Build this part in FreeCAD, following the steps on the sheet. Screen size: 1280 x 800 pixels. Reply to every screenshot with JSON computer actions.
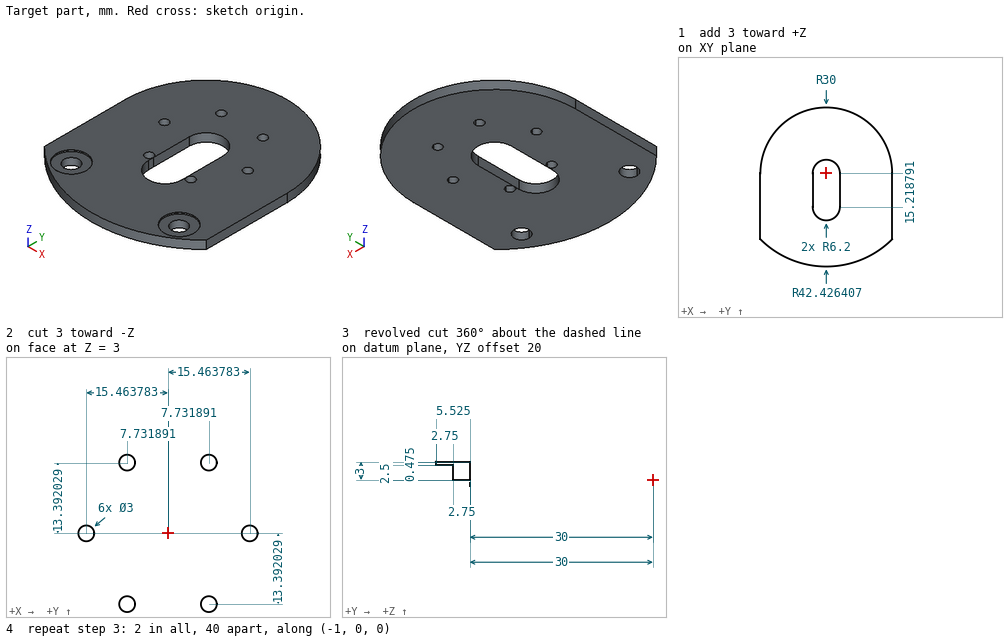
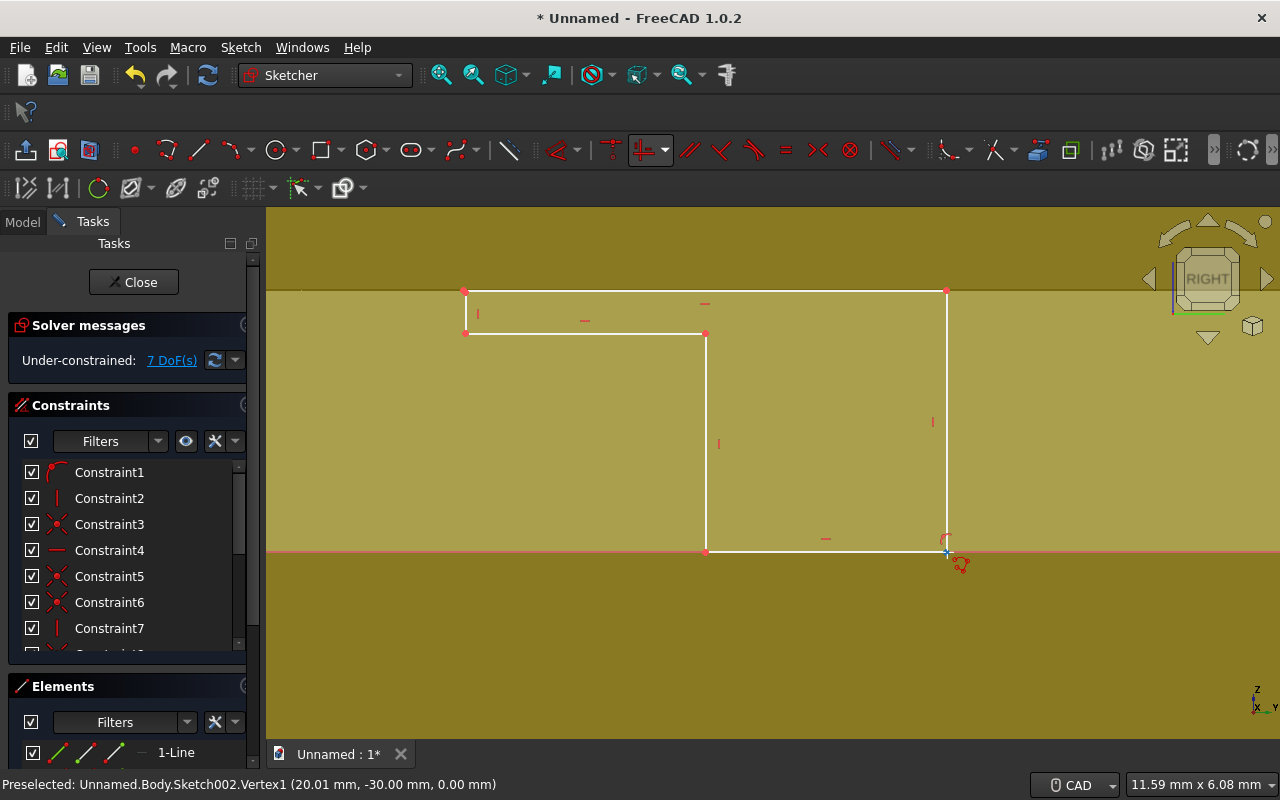
{"action": "key", "text": "g l"}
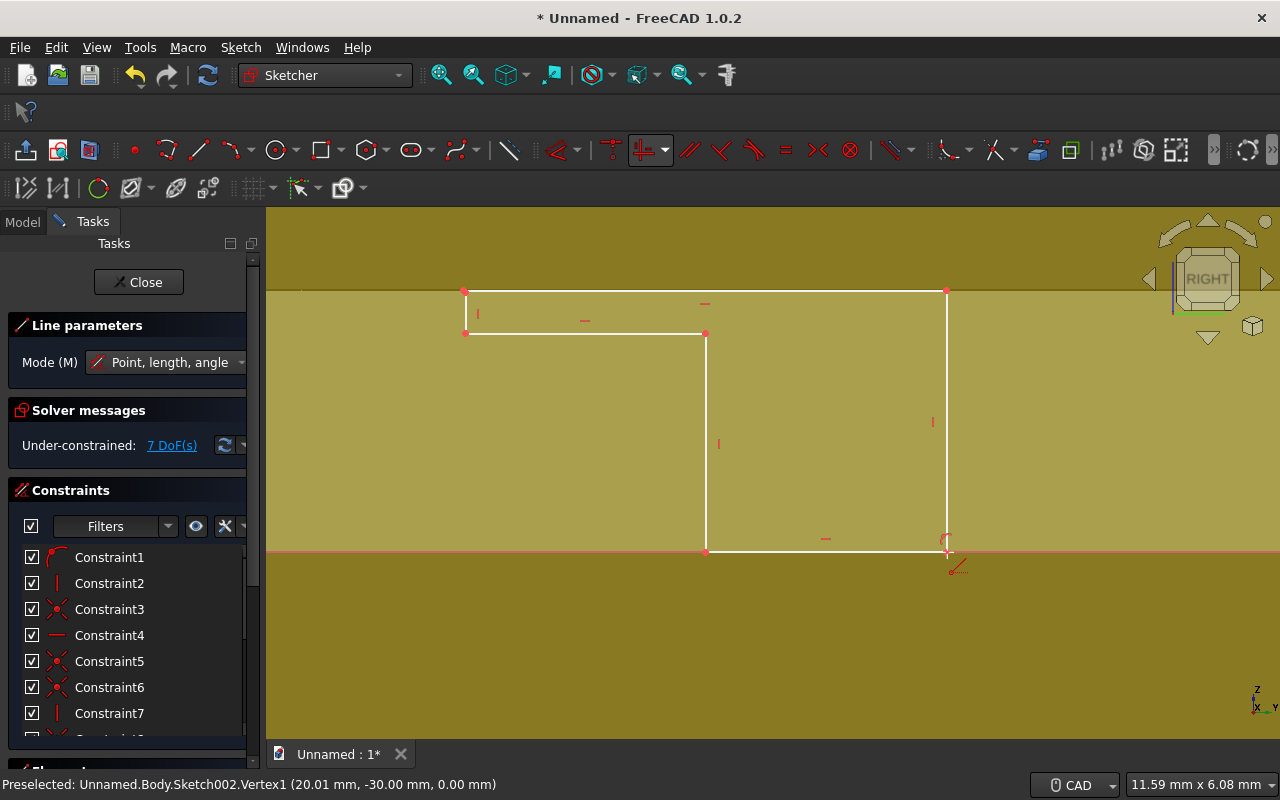
{"action": "left_click", "coordinate": [947, 578]}
{"action": "left_click", "coordinate": [947, 657]}
{"action": "key", "text": "Escape"}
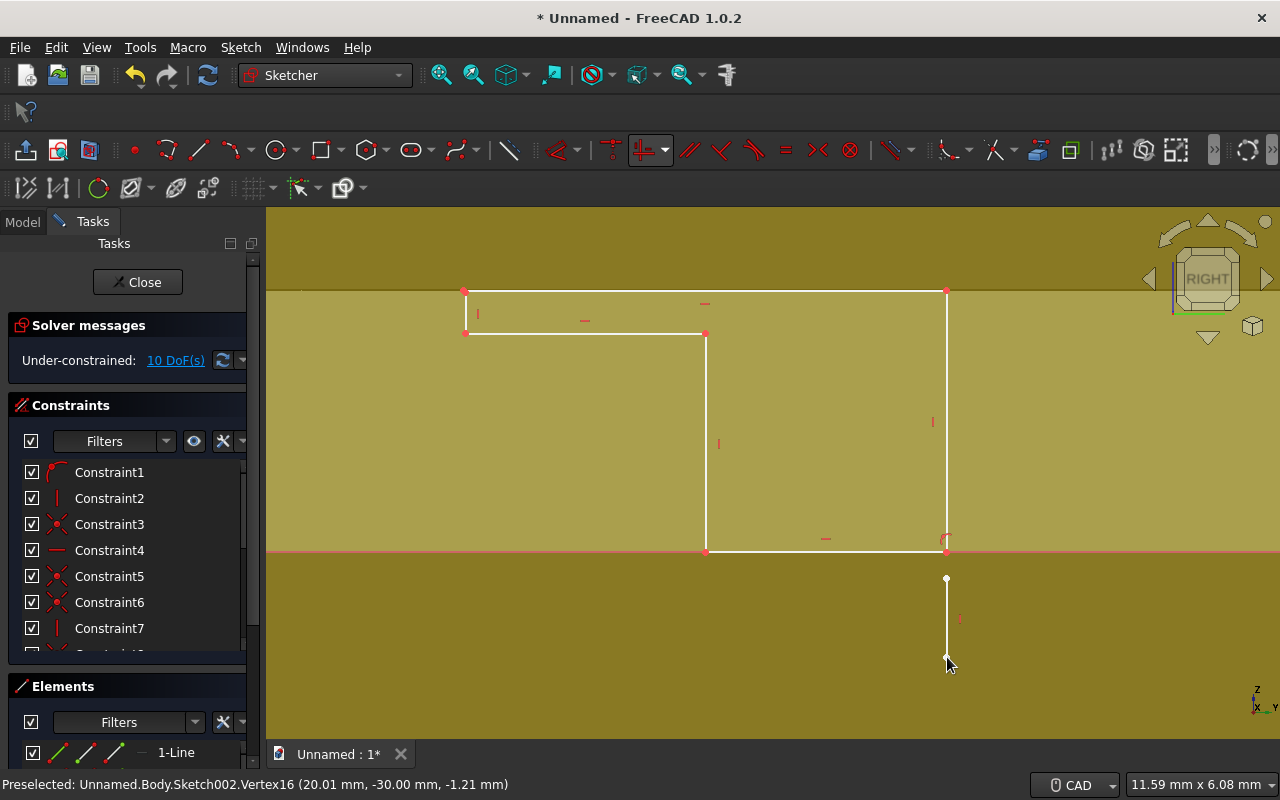
{"action": "left_click", "coordinate": [947, 603]}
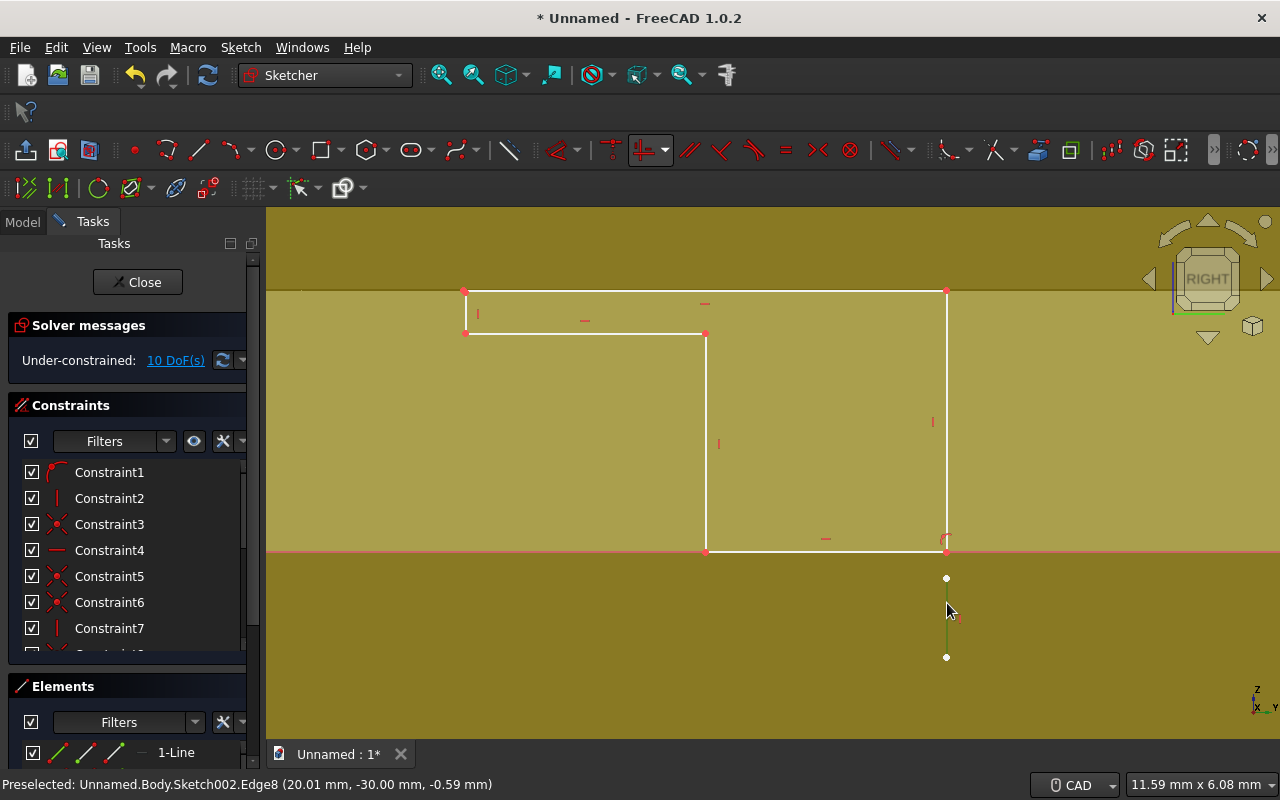
{"action": "key", "text": "g n"}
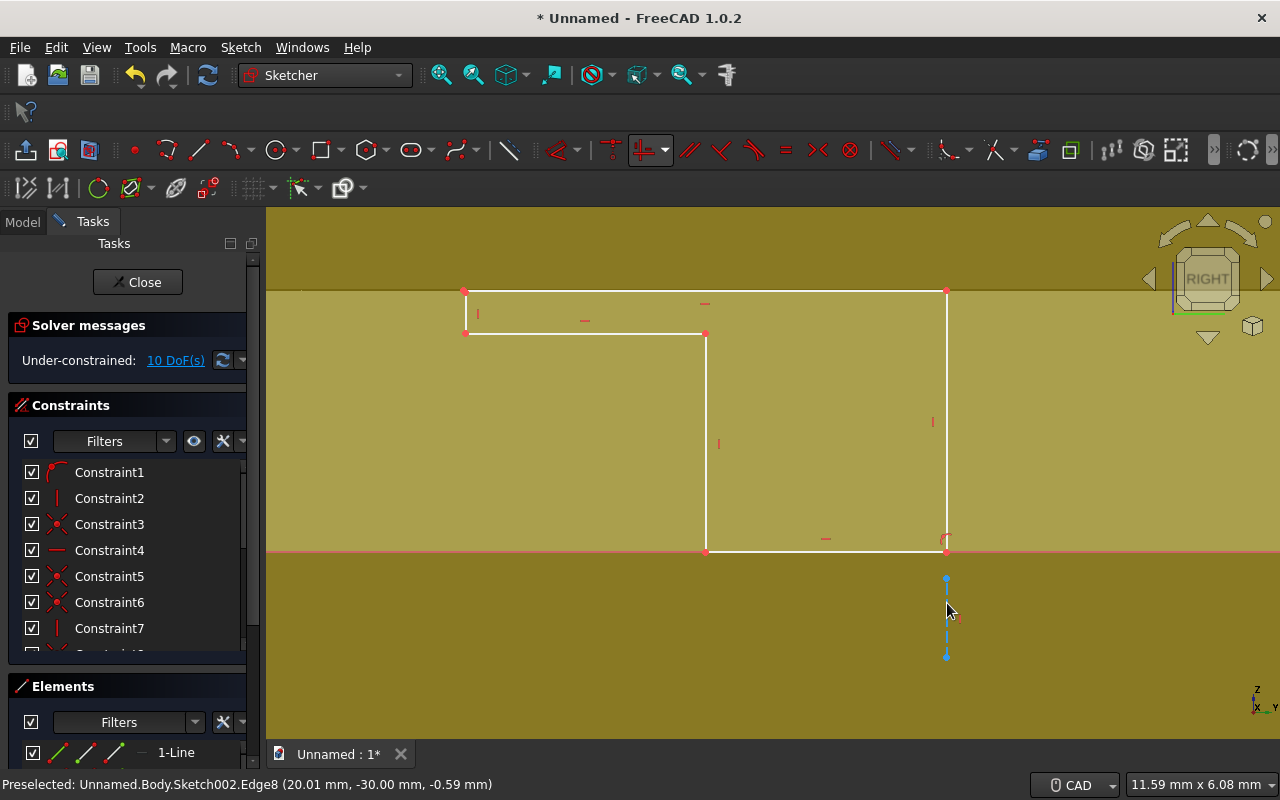
{"action": "key", "text": "d"}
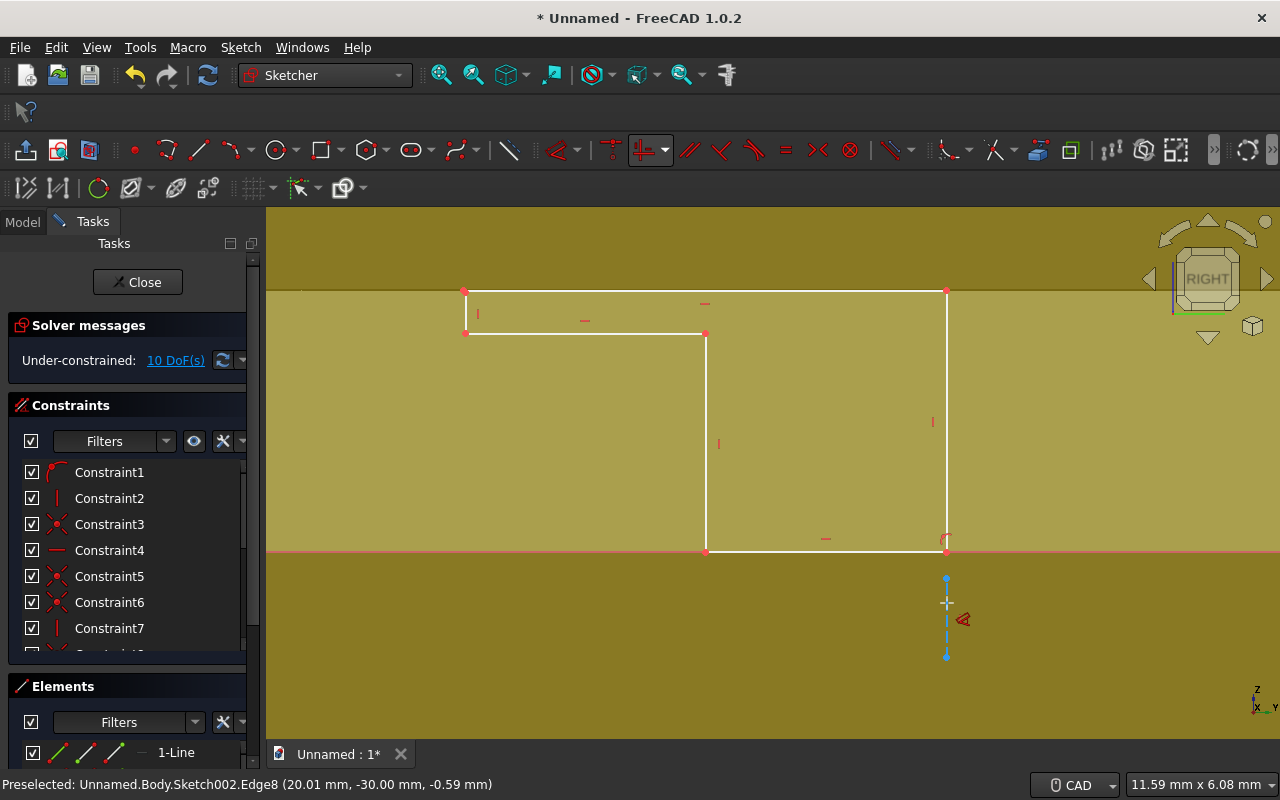
{"action": "left_click", "coordinate": [947, 474]}
{"action": "left_click", "coordinate": [981, 421]}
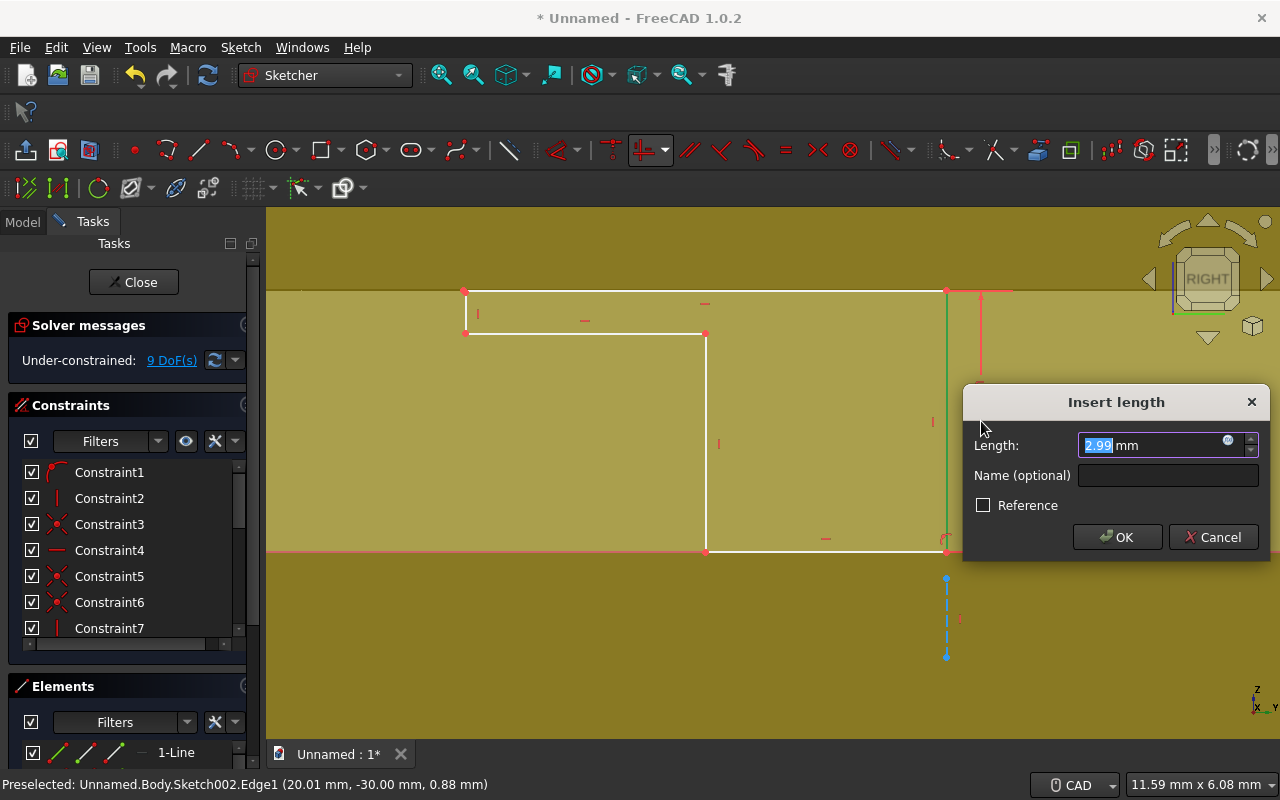
{"action": "type", "text": "3"}
{"action": "key", "text": "Return"}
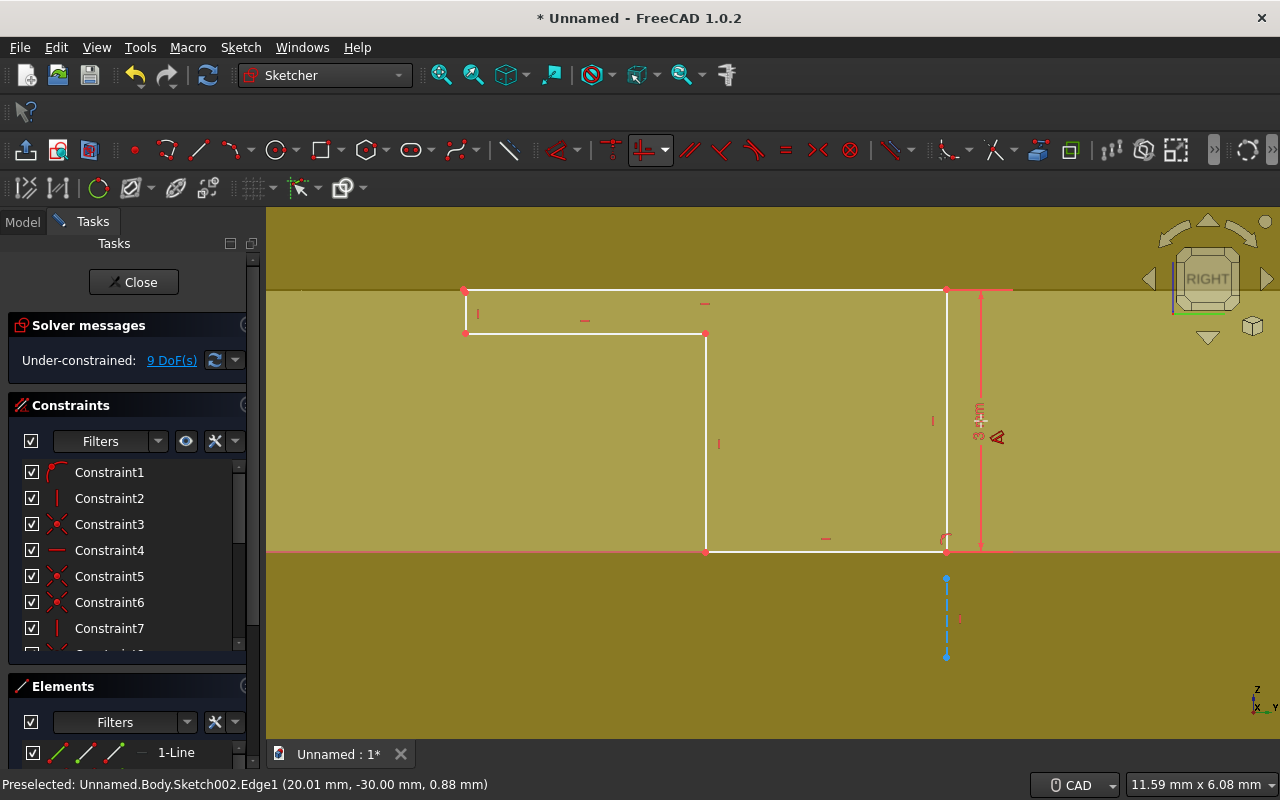
{"action": "left_click", "coordinate": [706, 399]}
{"action": "left_click", "coordinate": [740, 443]}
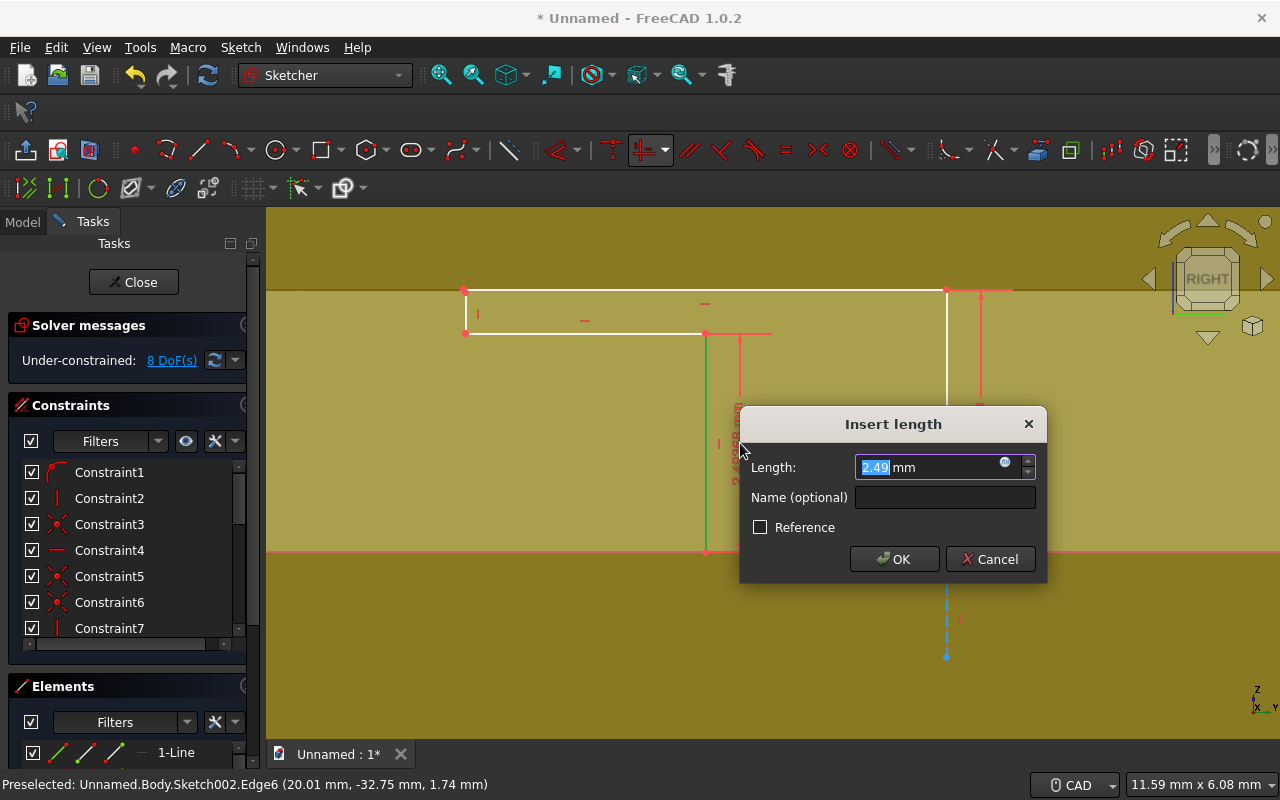
{"action": "type", "text": "2.5"}
{"action": "key", "text": "Return"}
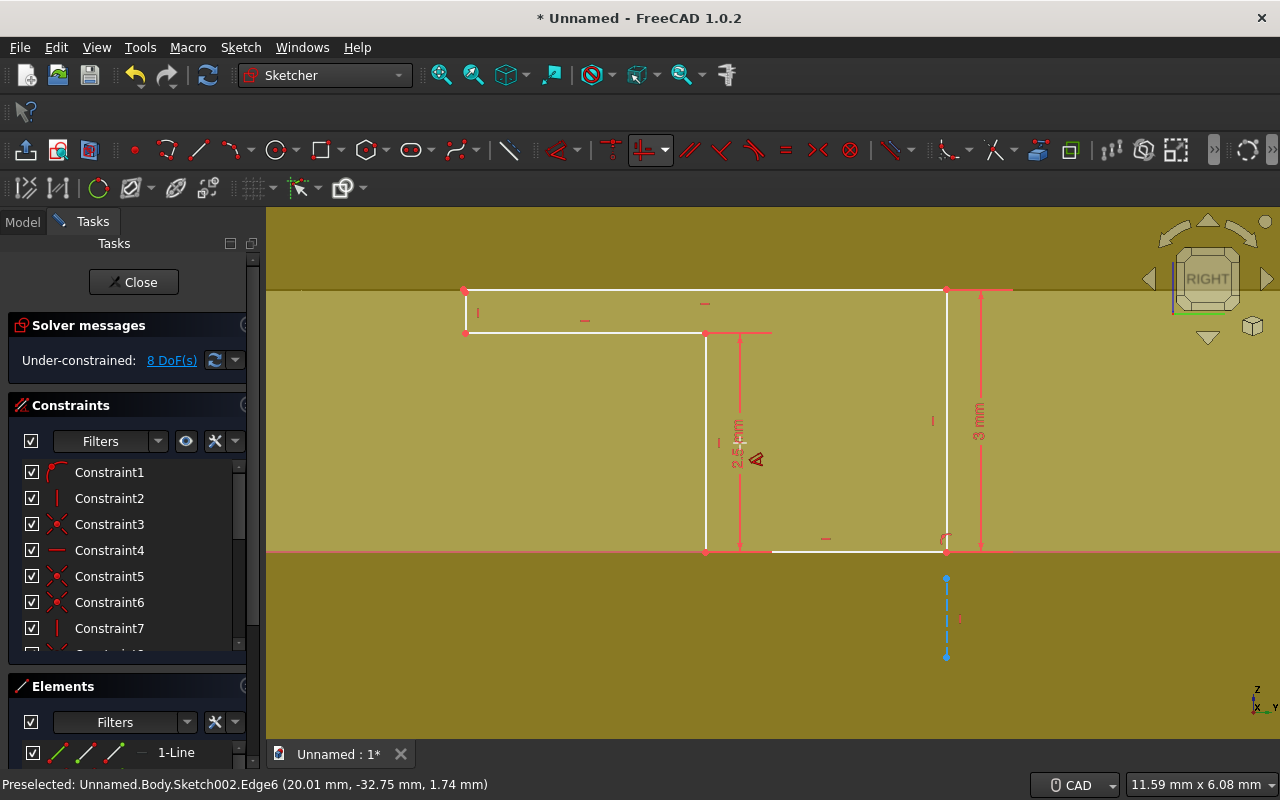
{"action": "left_click", "coordinate": [947, 552]}
{"action": "left_click", "coordinate": [1031, 586]}